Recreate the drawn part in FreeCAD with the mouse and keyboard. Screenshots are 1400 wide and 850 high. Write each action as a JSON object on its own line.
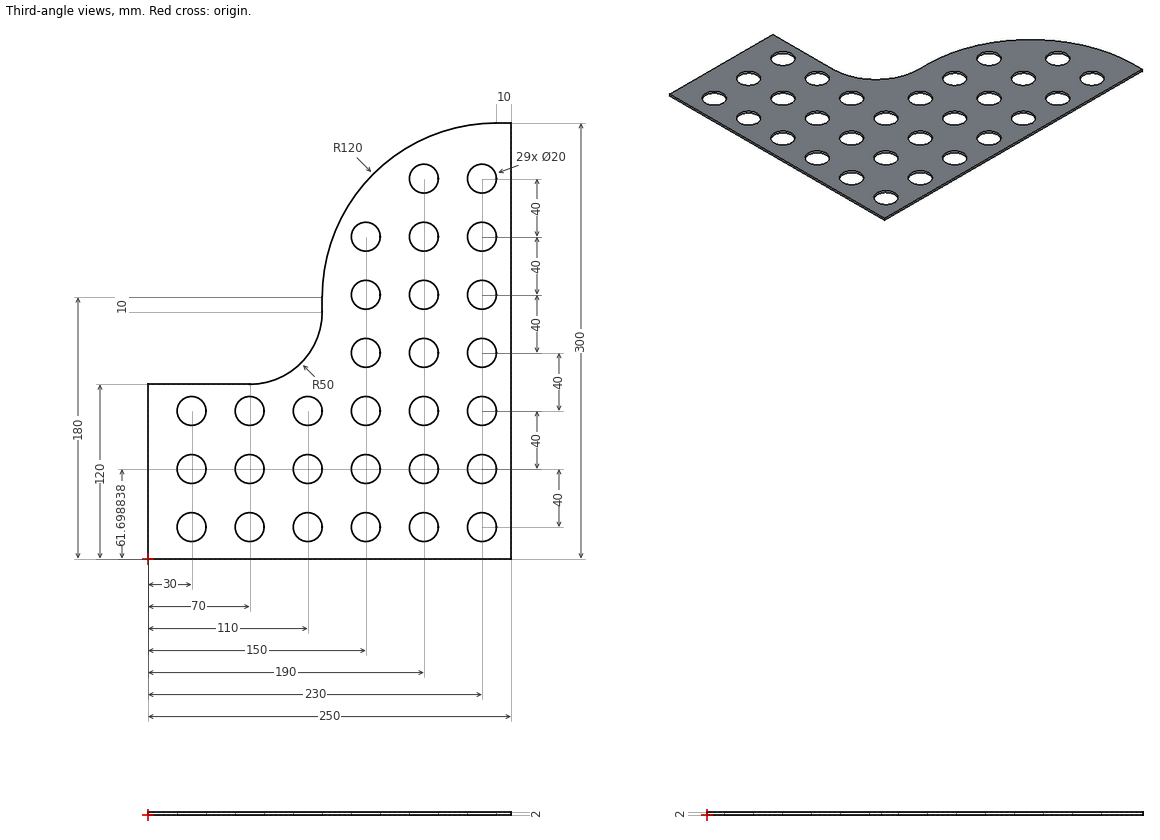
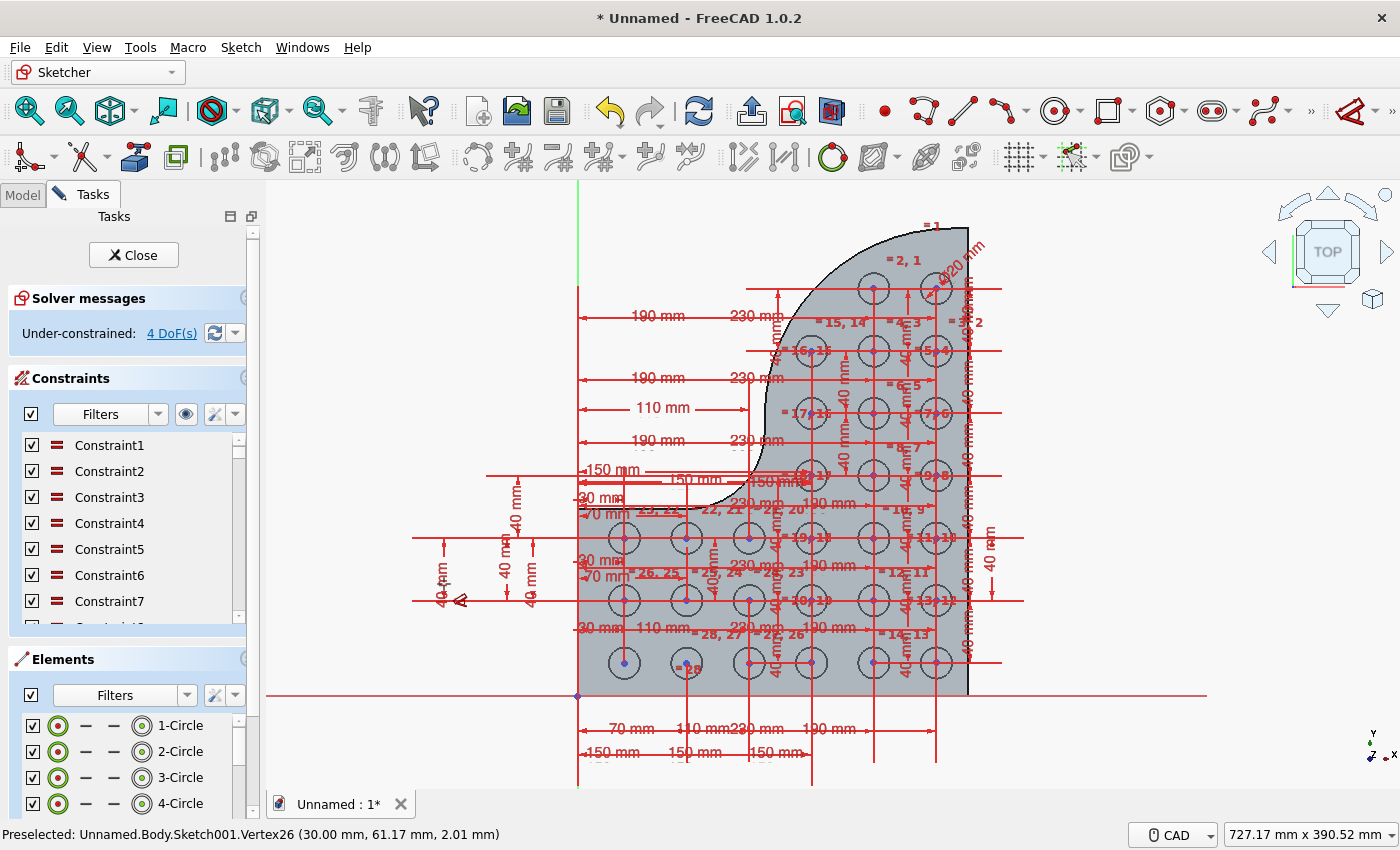
{"action": "left_click", "coordinate": [749, 601]}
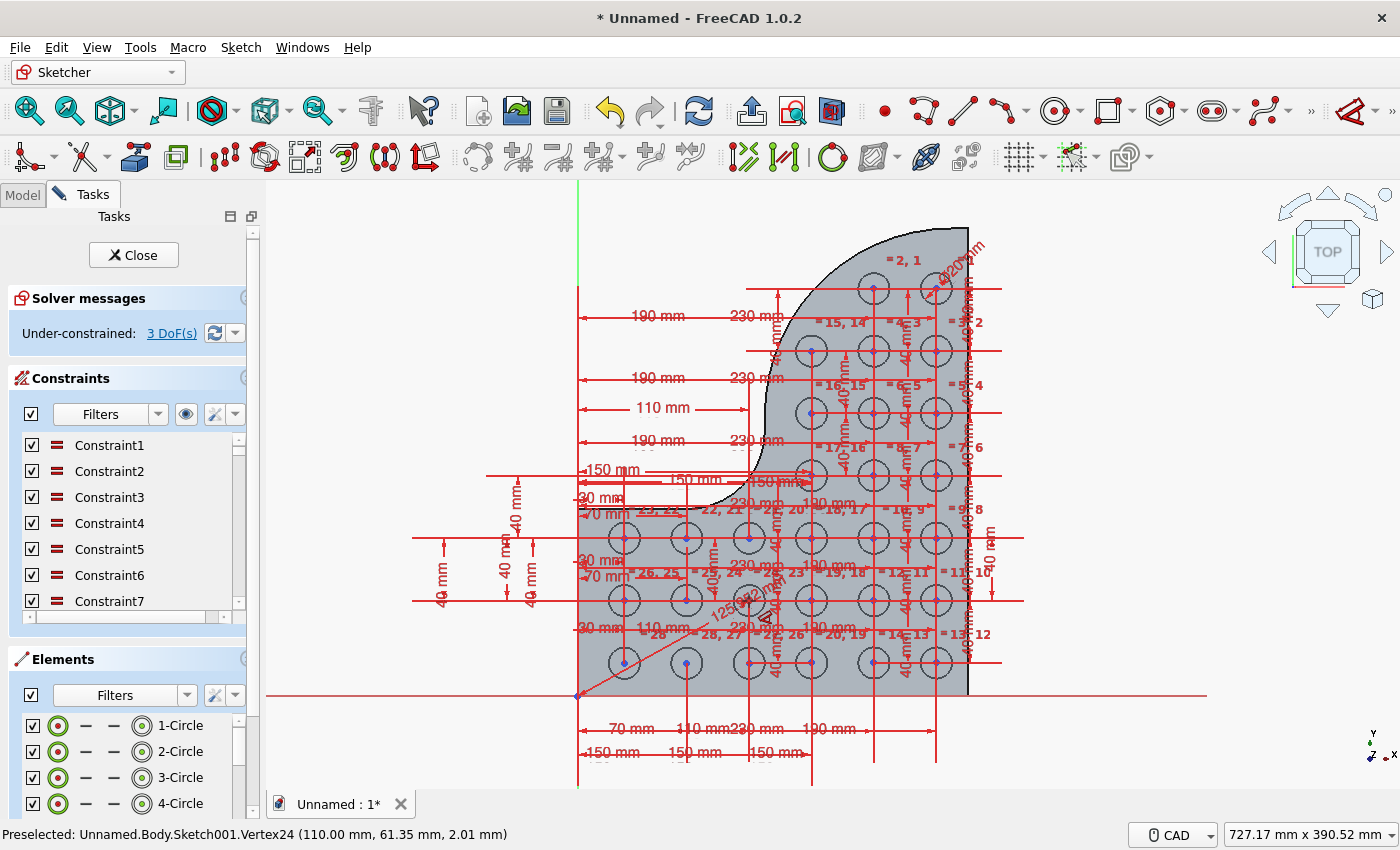
{"action": "left_click", "coordinate": [749, 663]}
{"action": "left_click", "coordinate": [595, 654]}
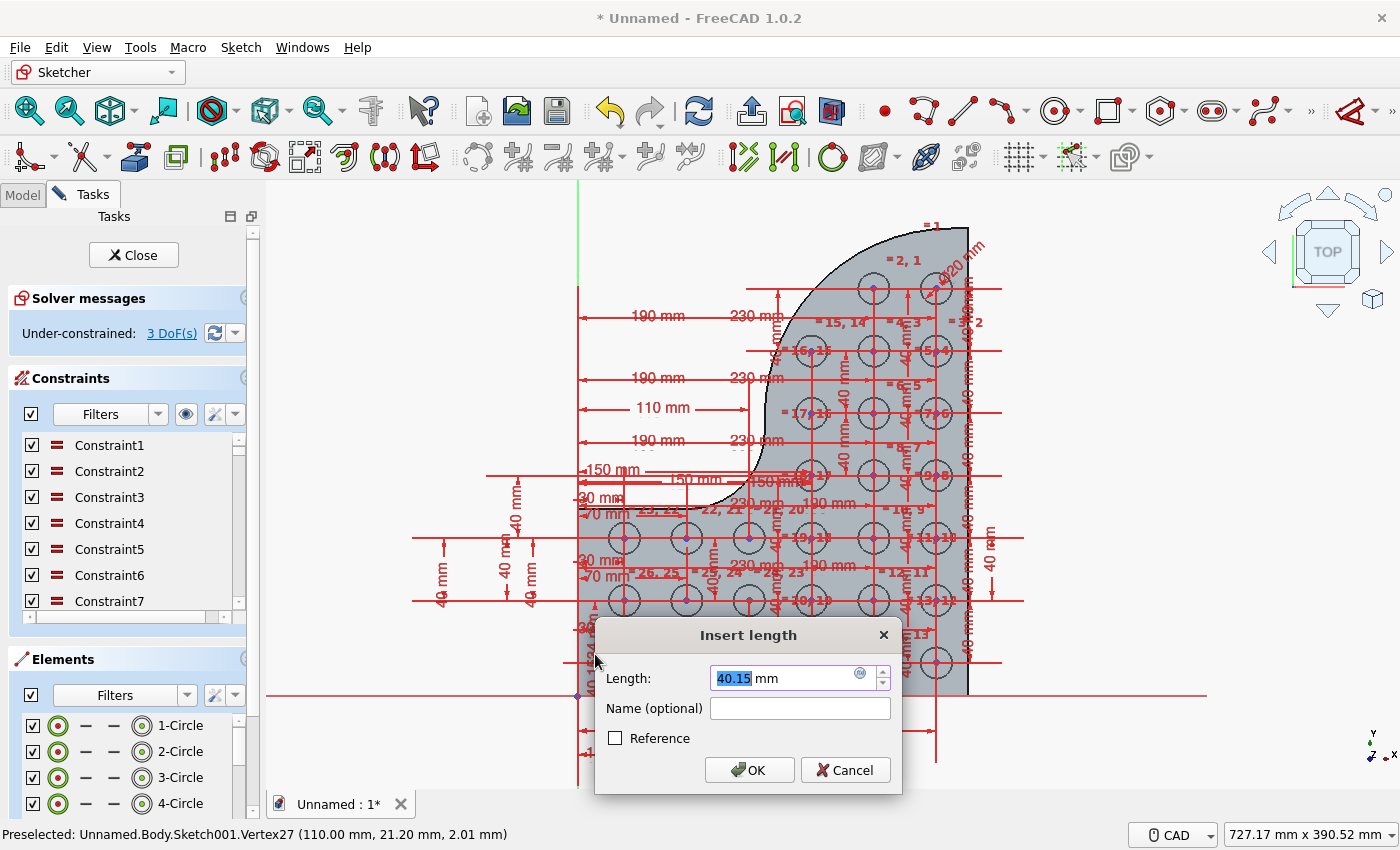
{"action": "type", "text": "40"}
{"action": "key", "text": "Return"}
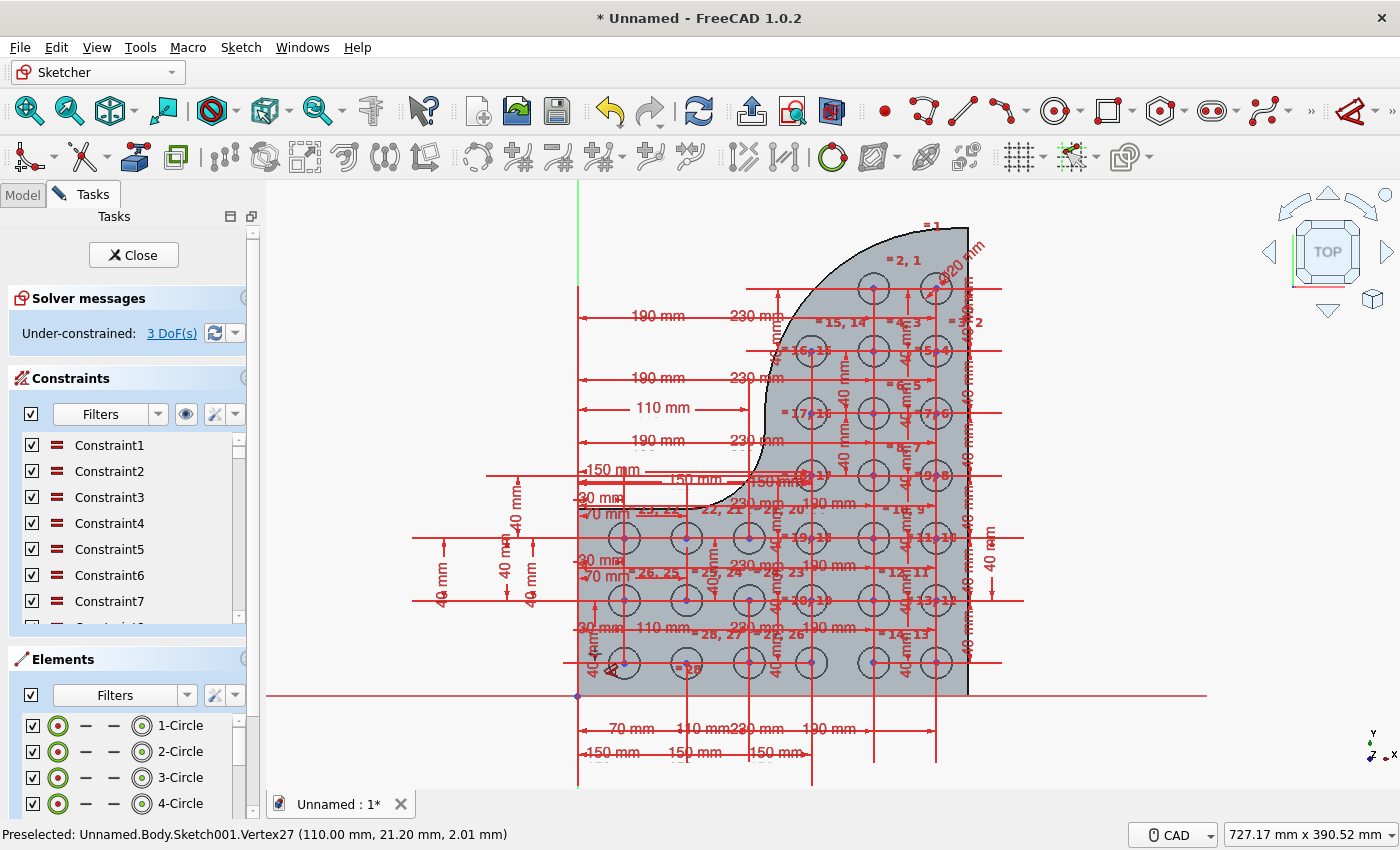
{"action": "left_click", "coordinate": [687, 601]}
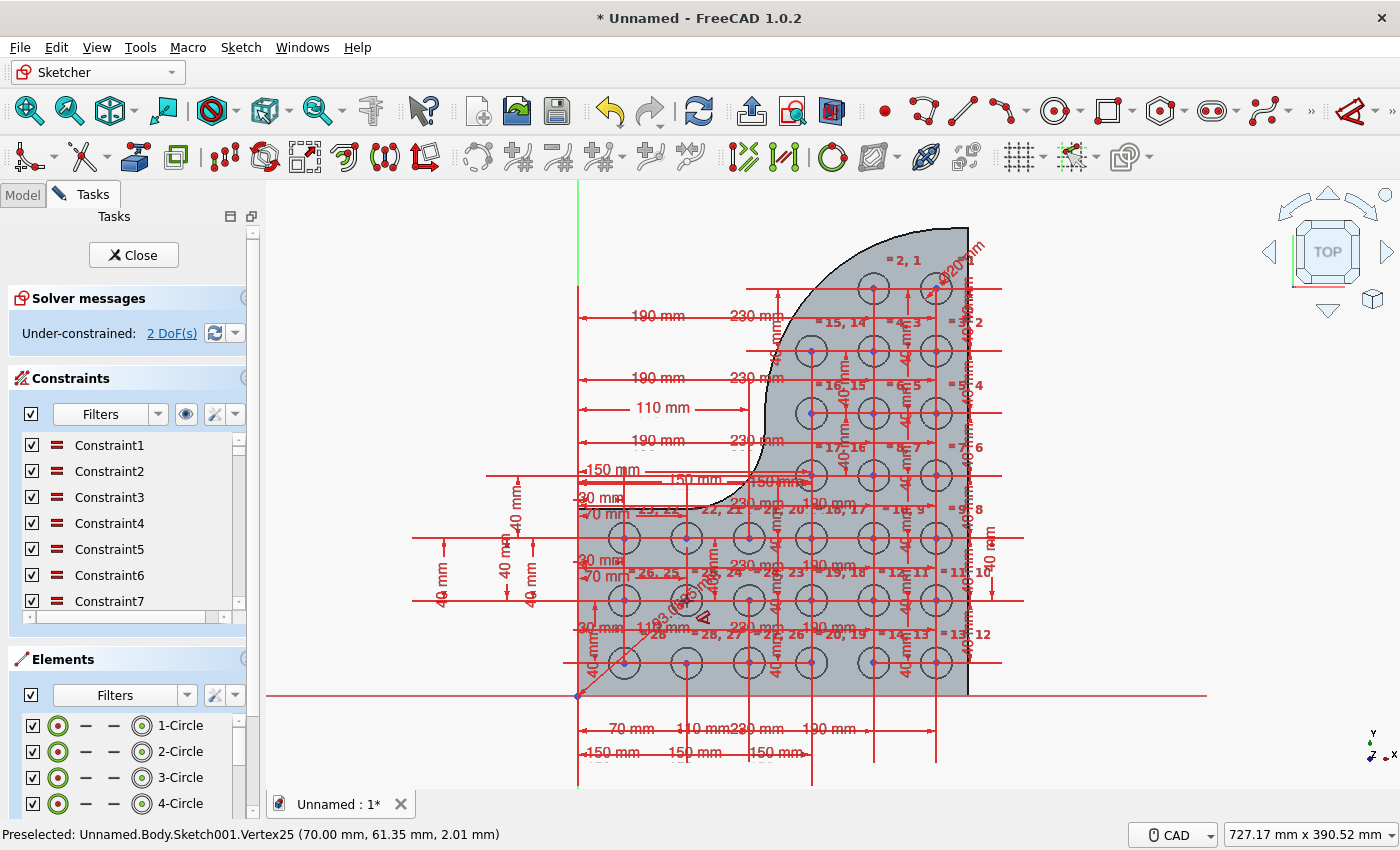
{"action": "left_click", "coordinate": [687, 663]}
{"action": "left_click", "coordinate": [507, 632]}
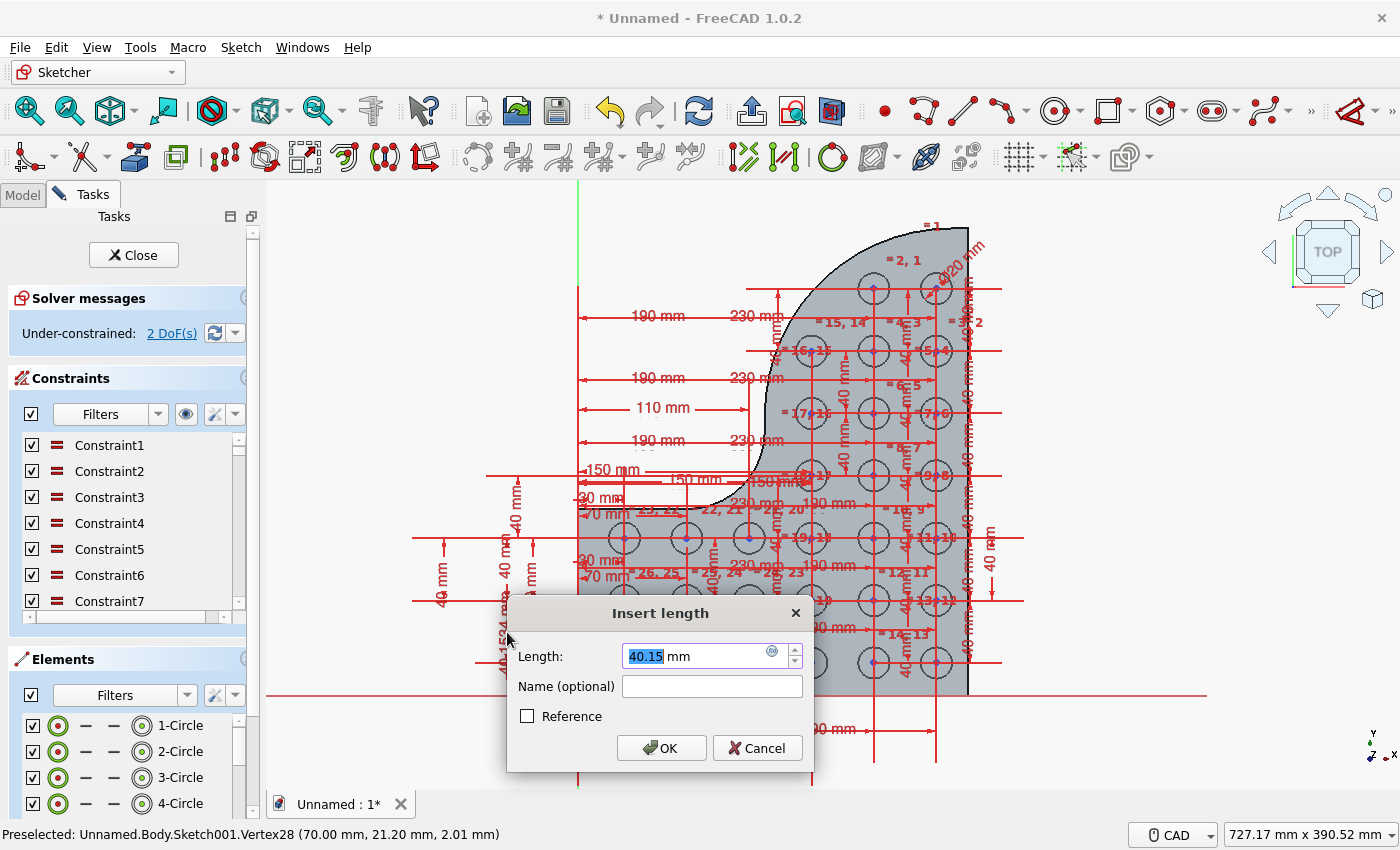
{"action": "type", "text": "40"}
{"action": "key", "text": "Return"}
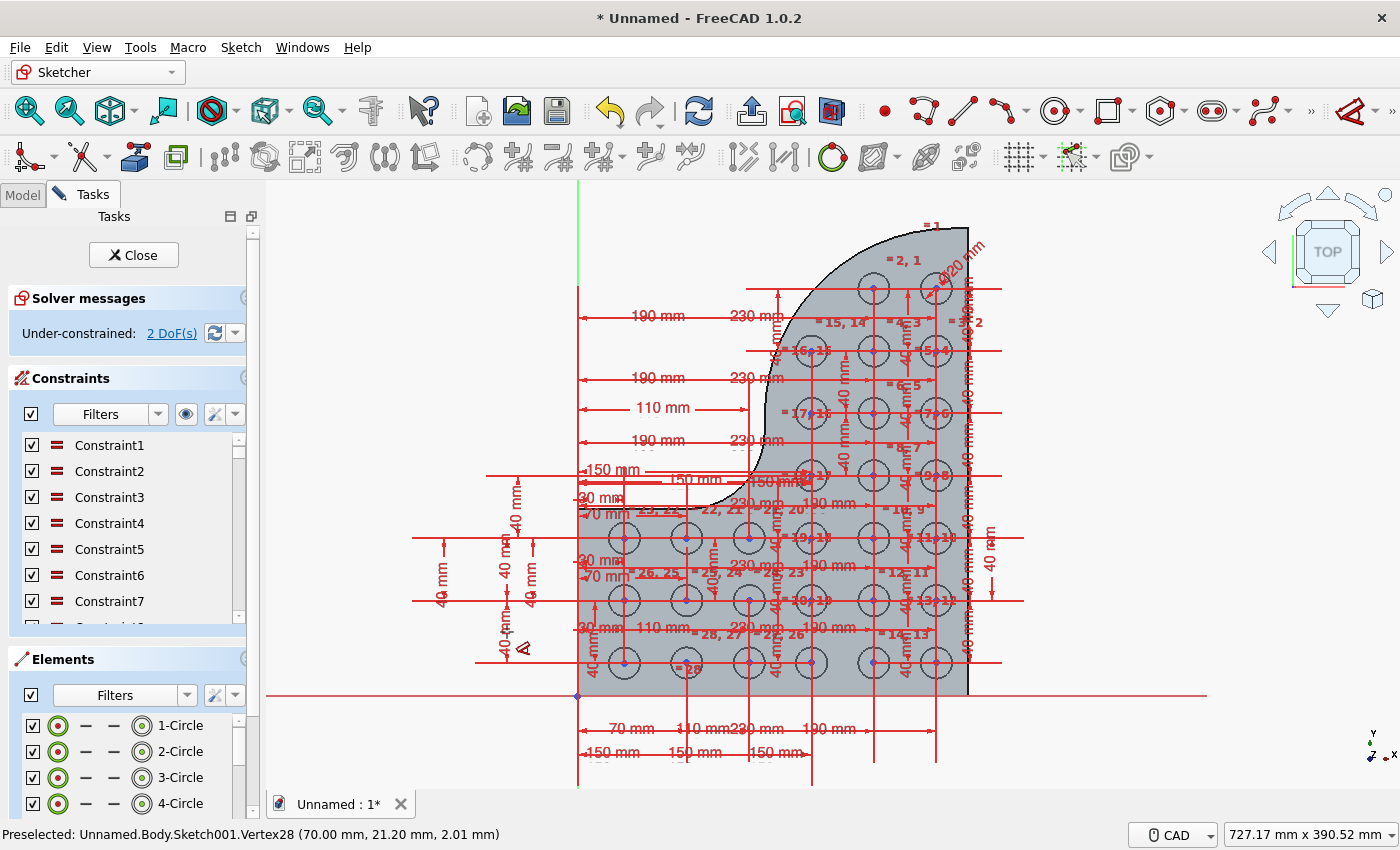
{"action": "left_click", "coordinate": [624, 601]}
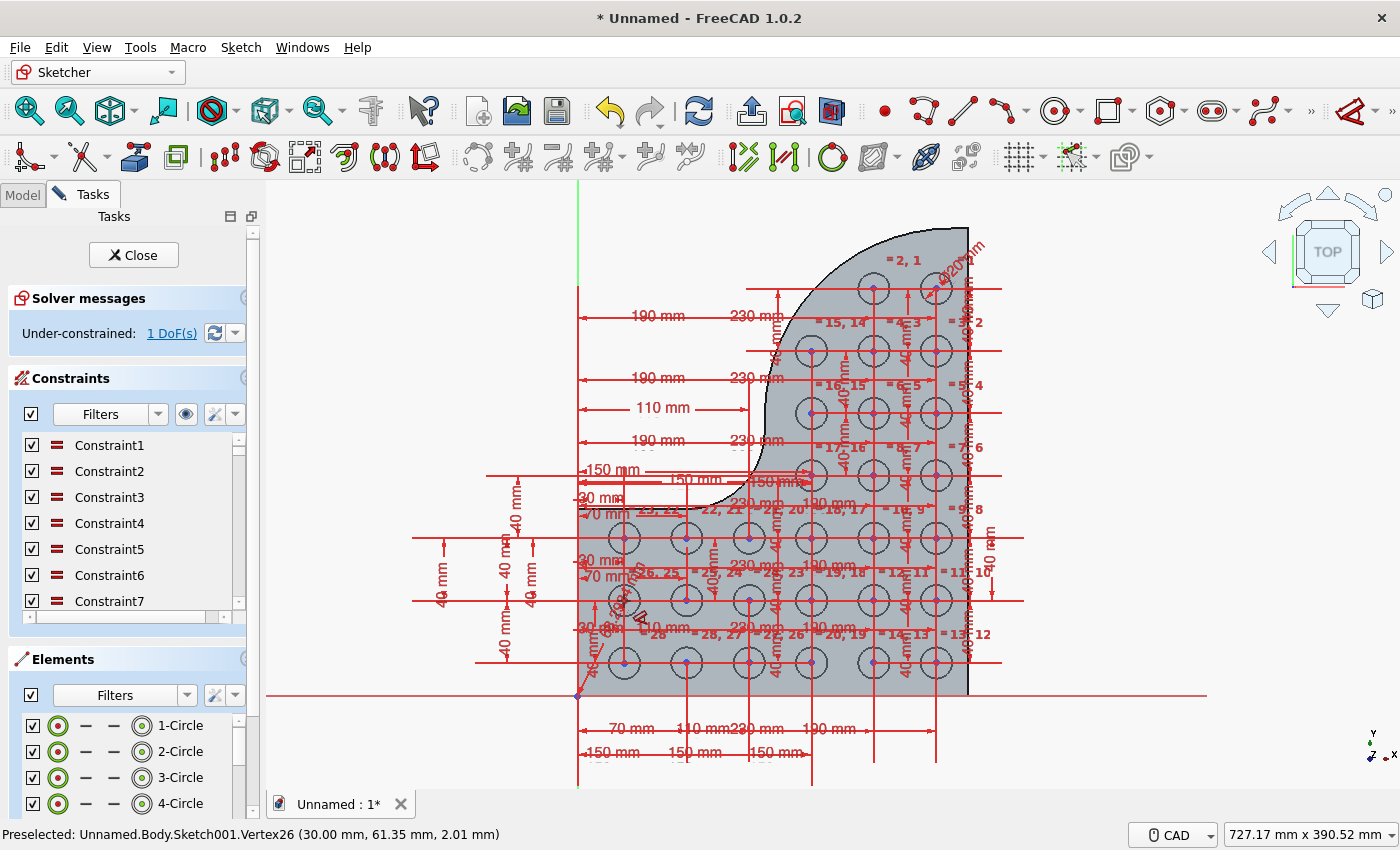
{"action": "left_click", "coordinate": [624, 663]}
{"action": "left_click", "coordinate": [518, 610]}